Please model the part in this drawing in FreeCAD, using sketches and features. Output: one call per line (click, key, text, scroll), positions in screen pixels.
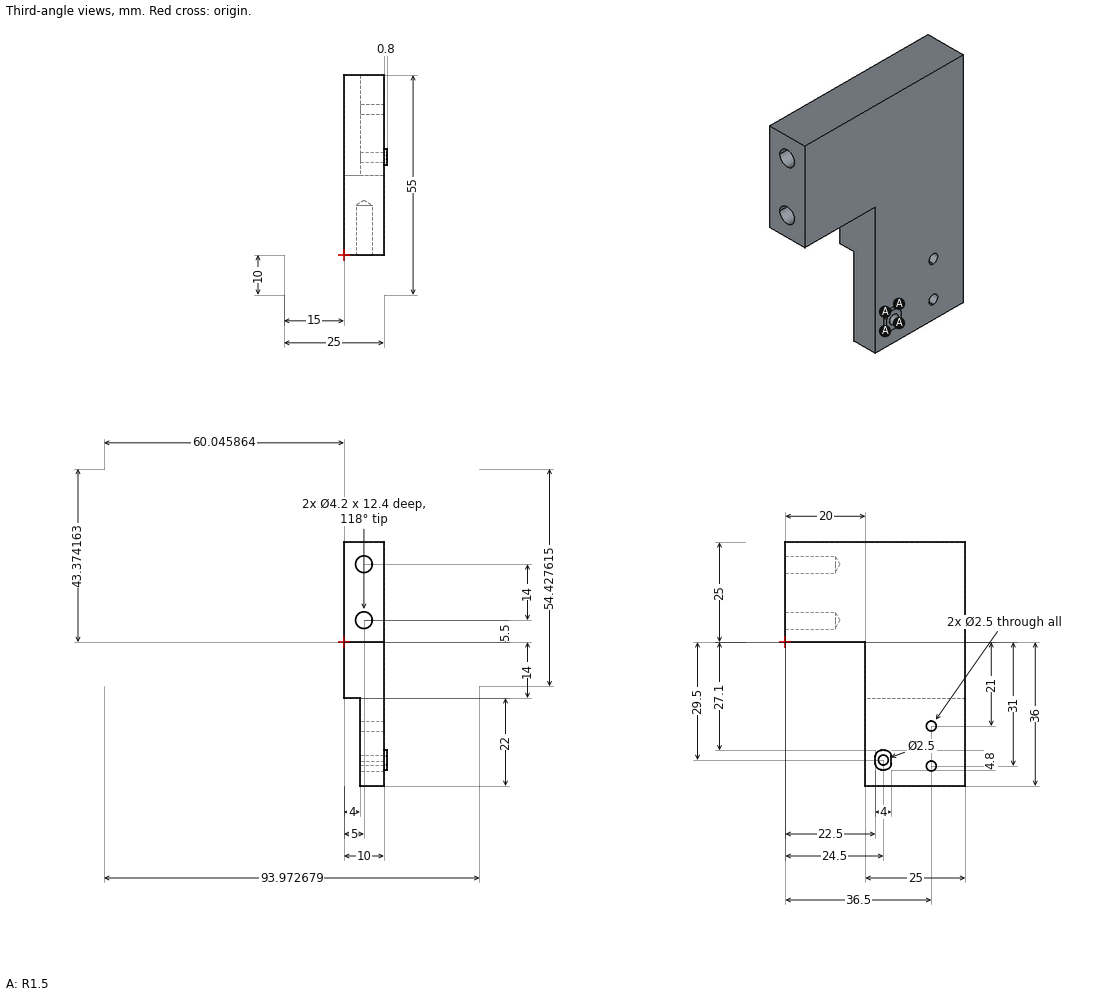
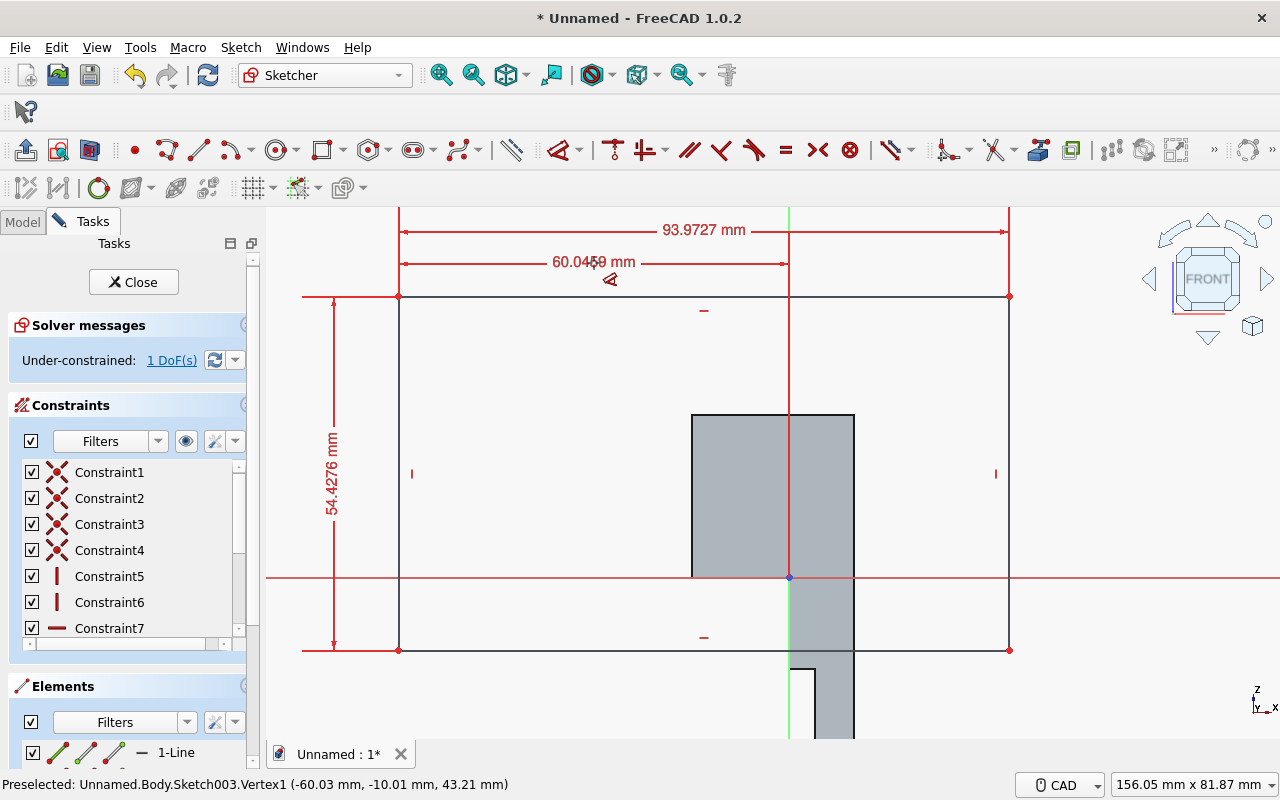
click(399, 297)
click(365, 437)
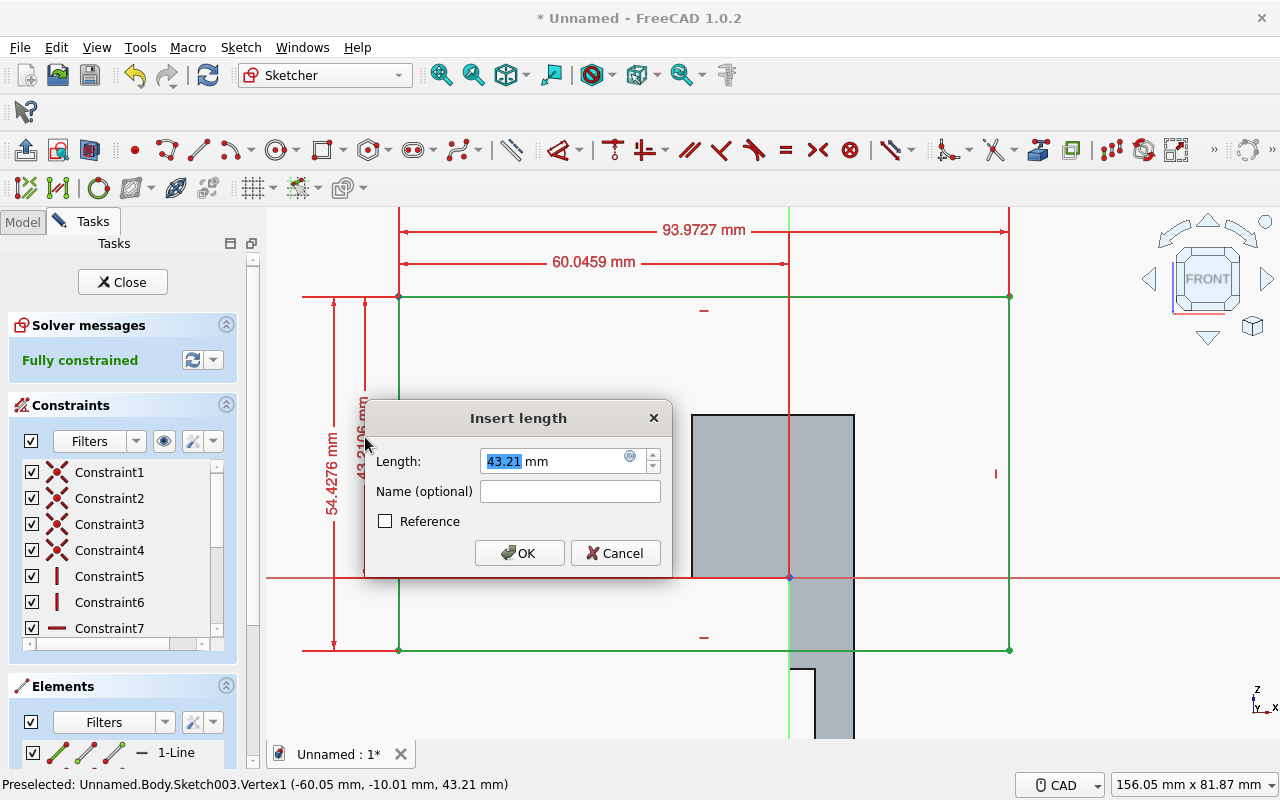
text(43.374163)
key(Return)
key(Escape)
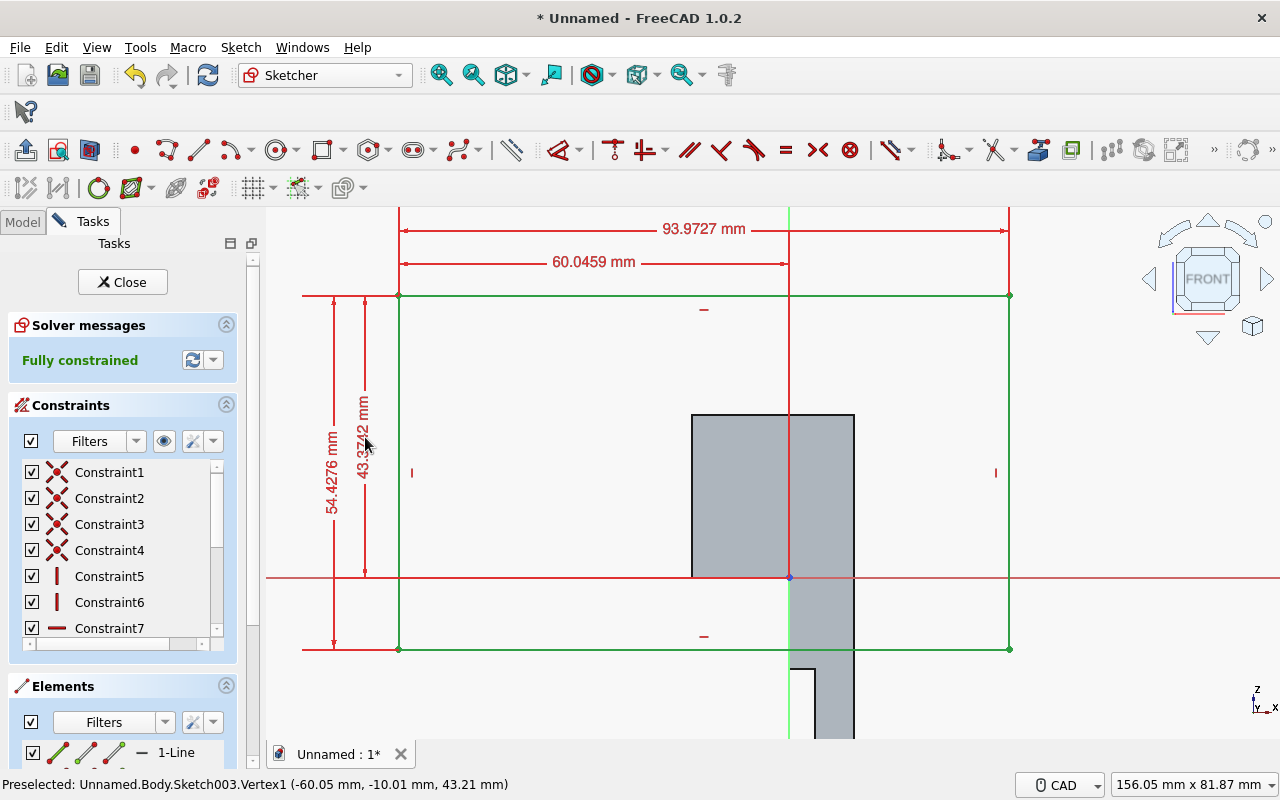
click(123, 282)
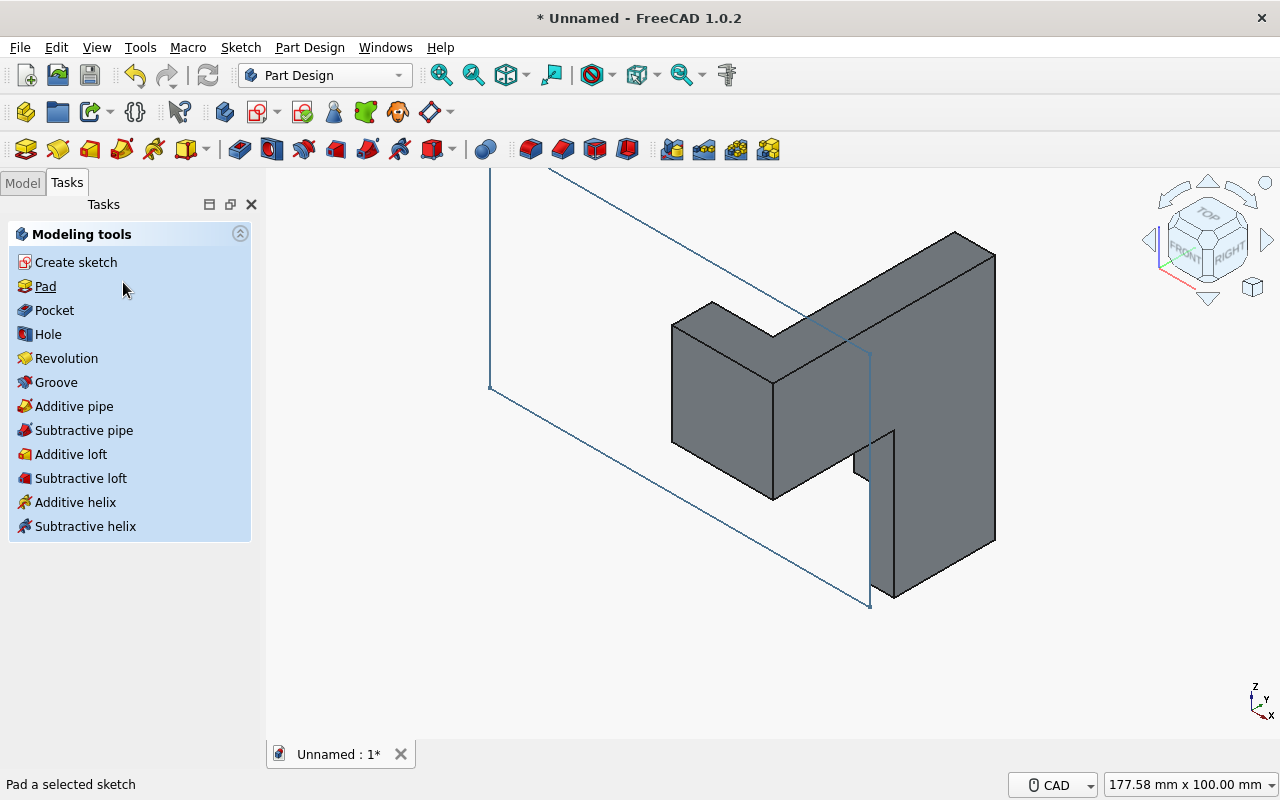
click(240, 150)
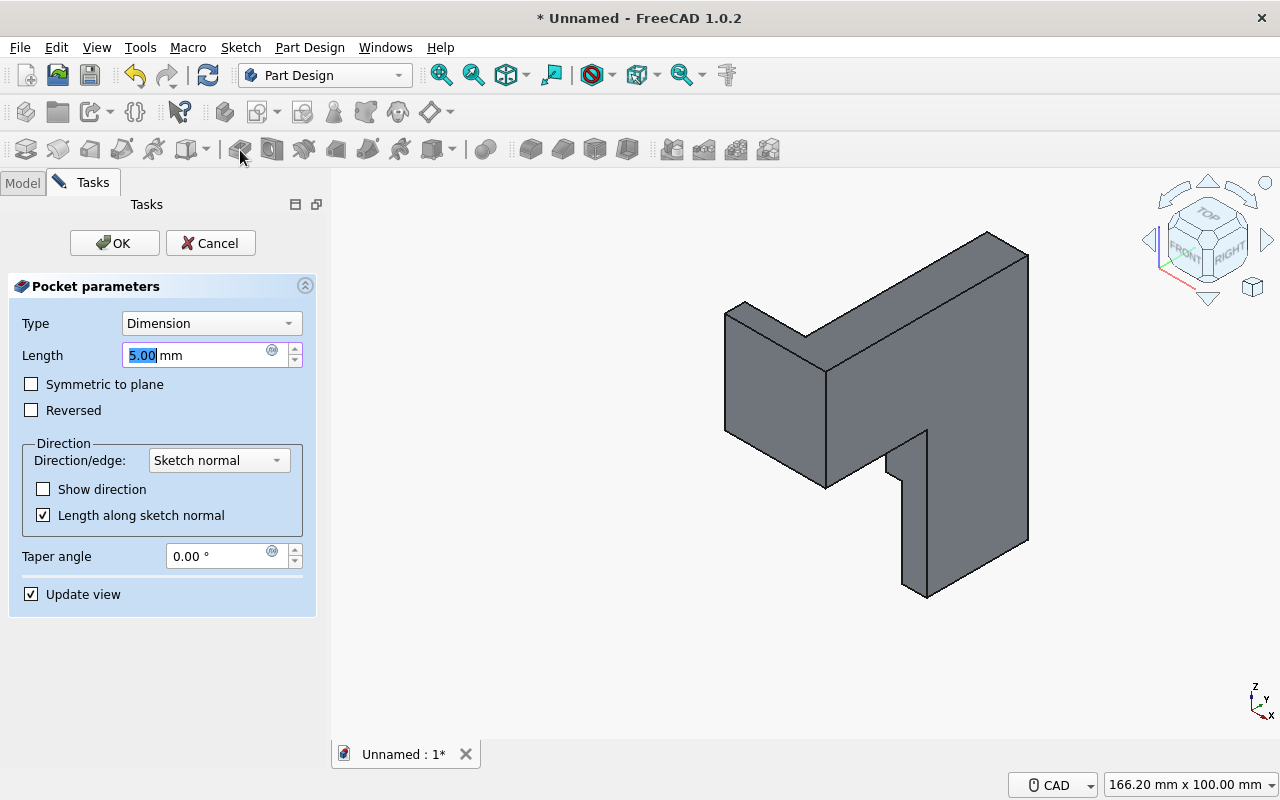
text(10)
key(Tab)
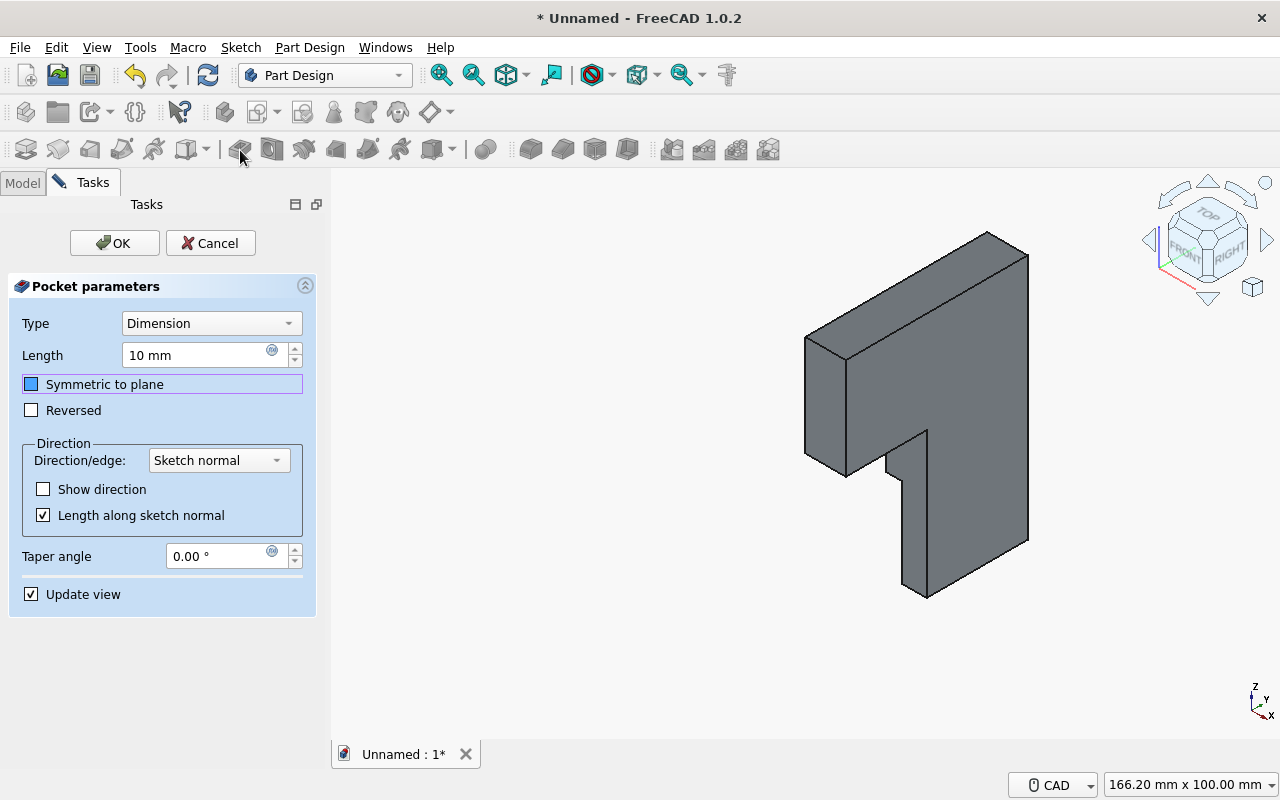
click(115, 243)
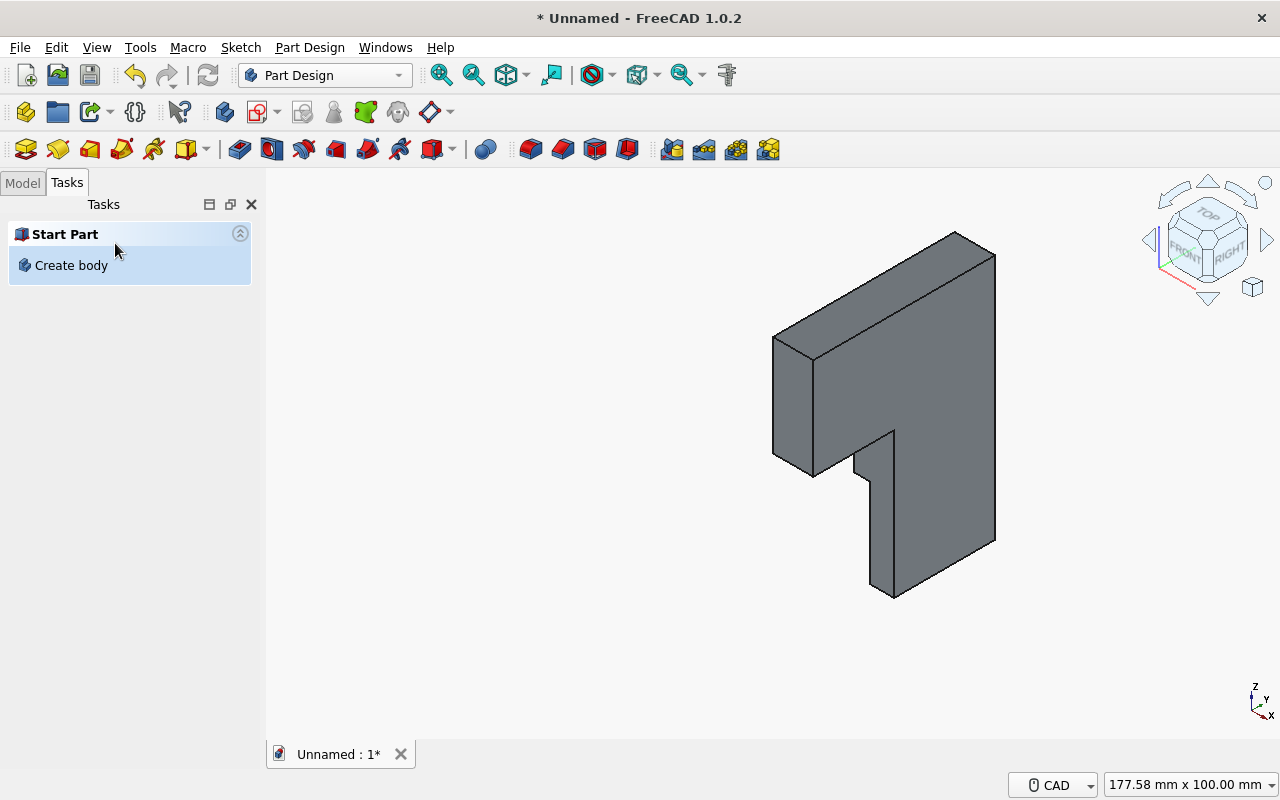
click(258, 112)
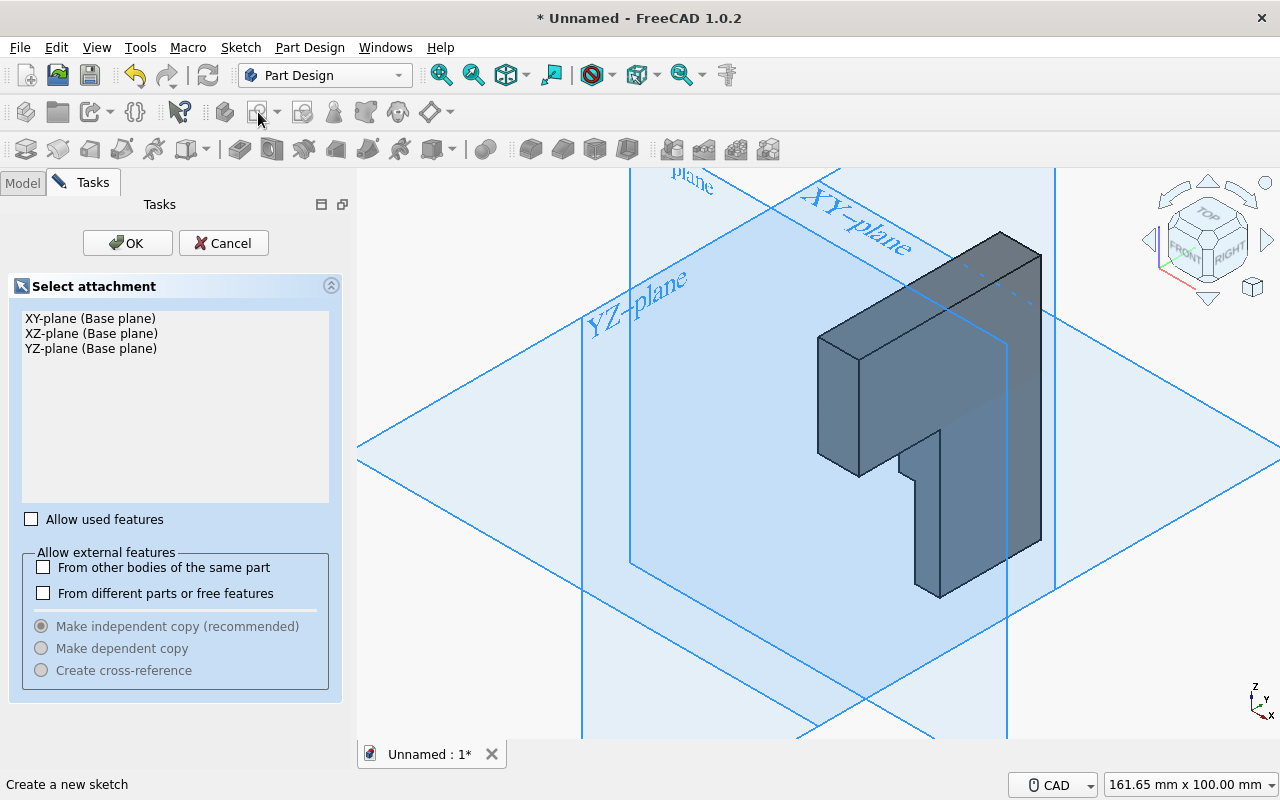
click(82, 334)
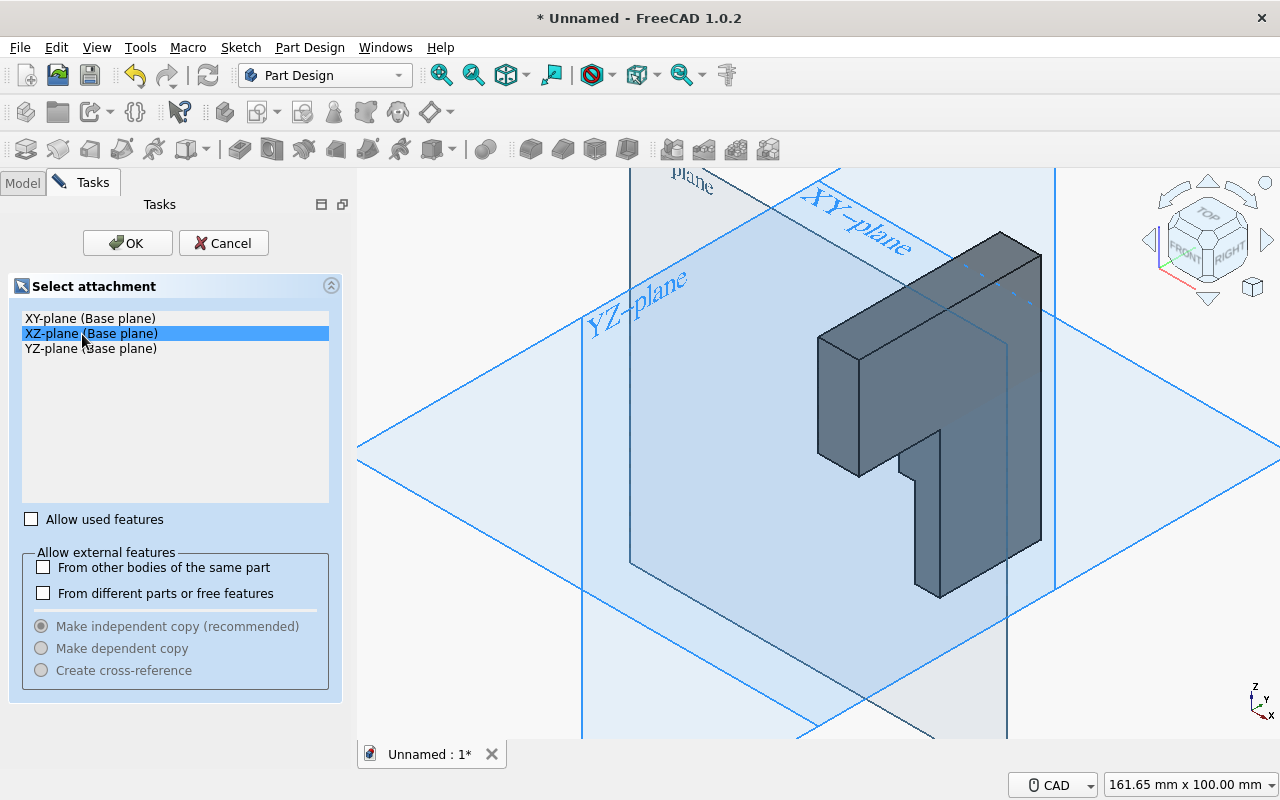
click(128, 243)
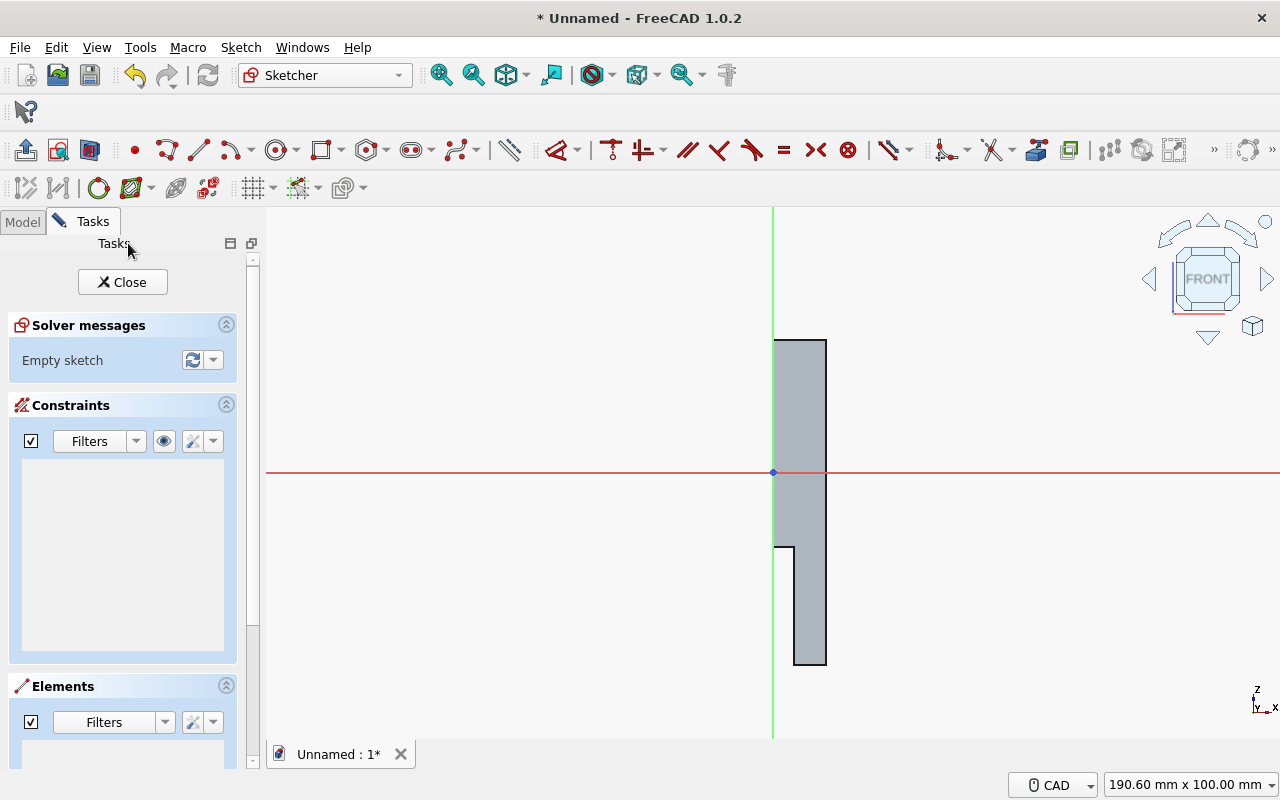
scroll(843, 382, up, 5)